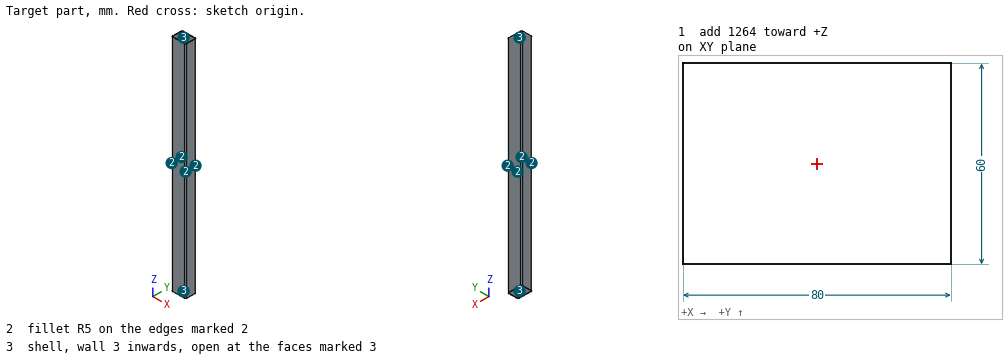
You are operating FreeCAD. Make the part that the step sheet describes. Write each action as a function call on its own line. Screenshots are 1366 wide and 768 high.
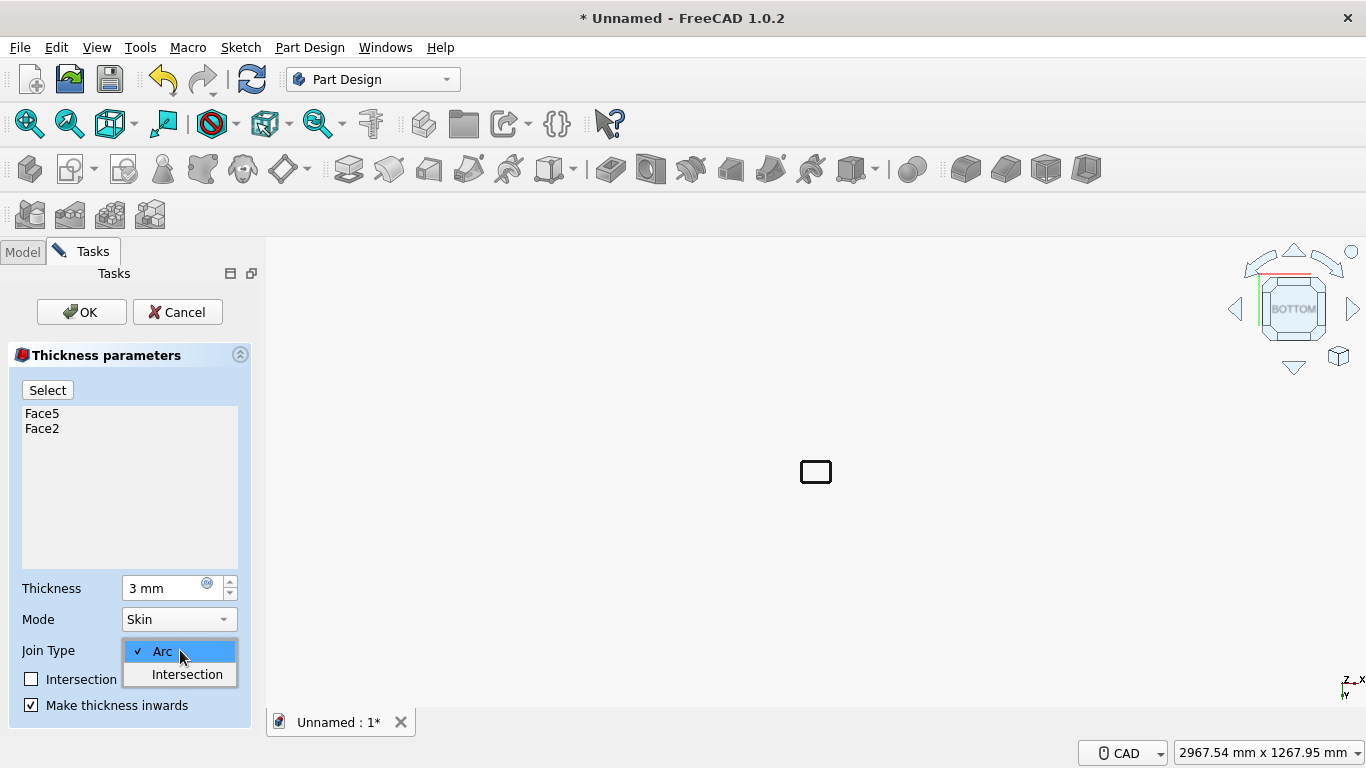
click(179, 674)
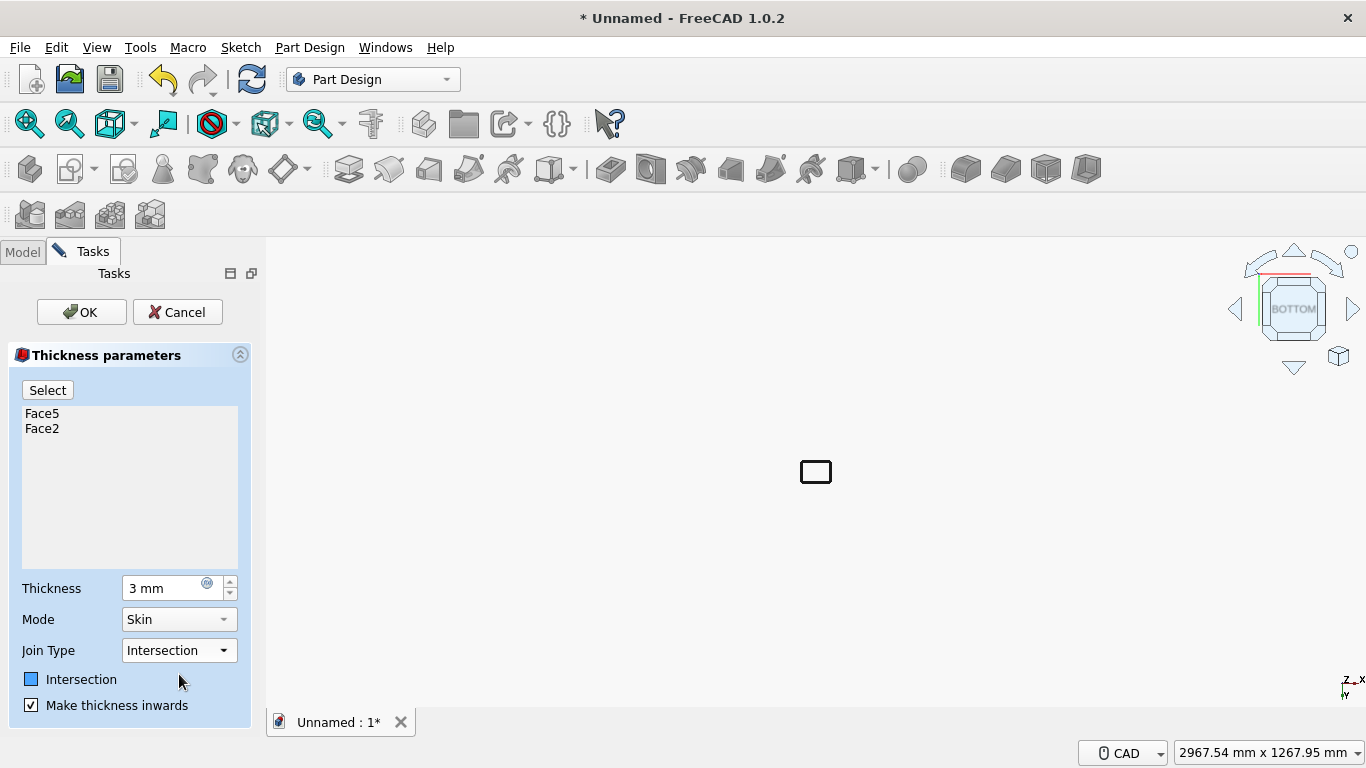
click(82, 312)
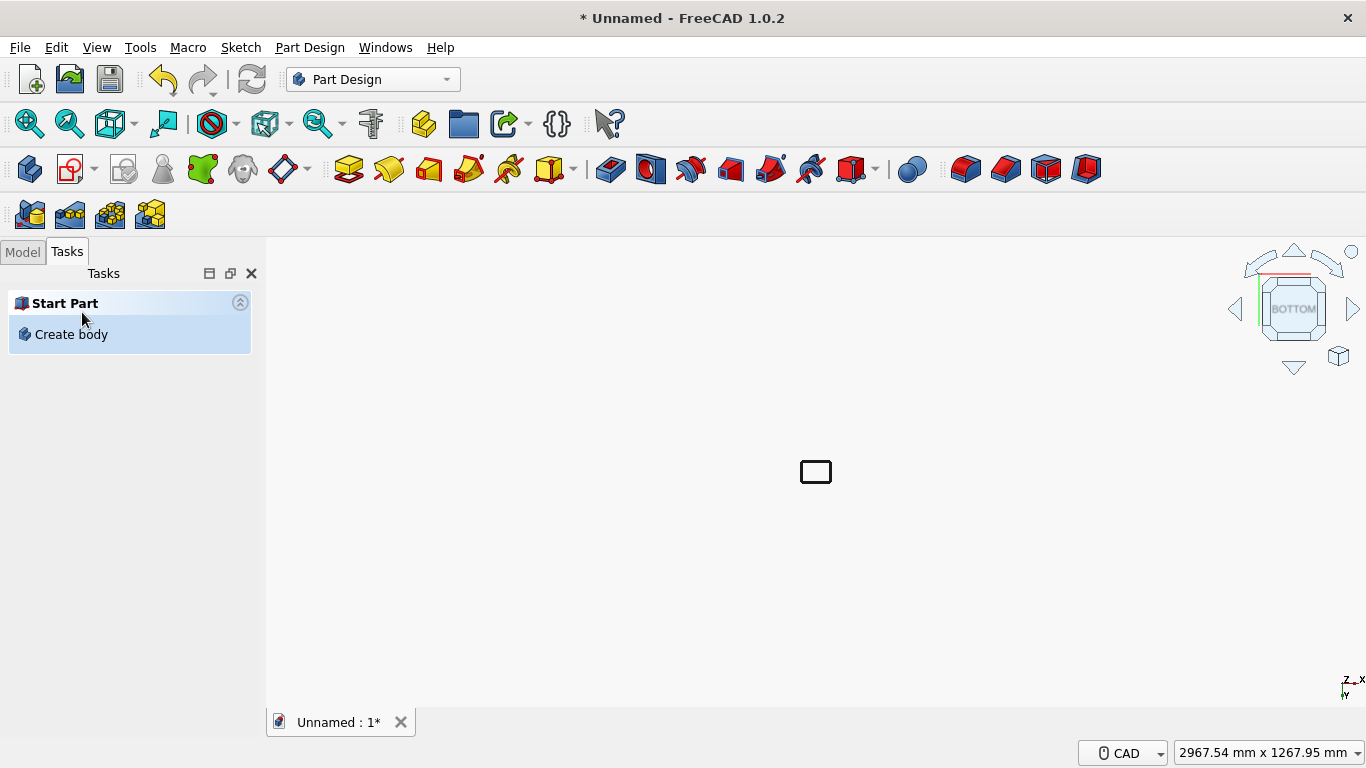
key(0)